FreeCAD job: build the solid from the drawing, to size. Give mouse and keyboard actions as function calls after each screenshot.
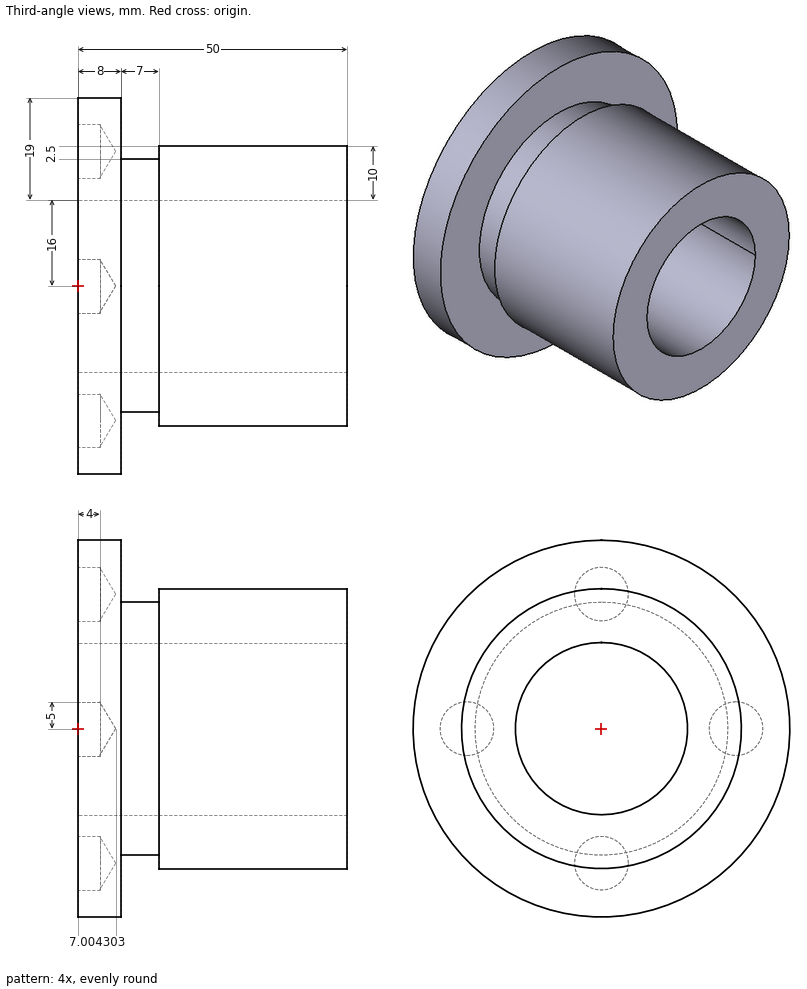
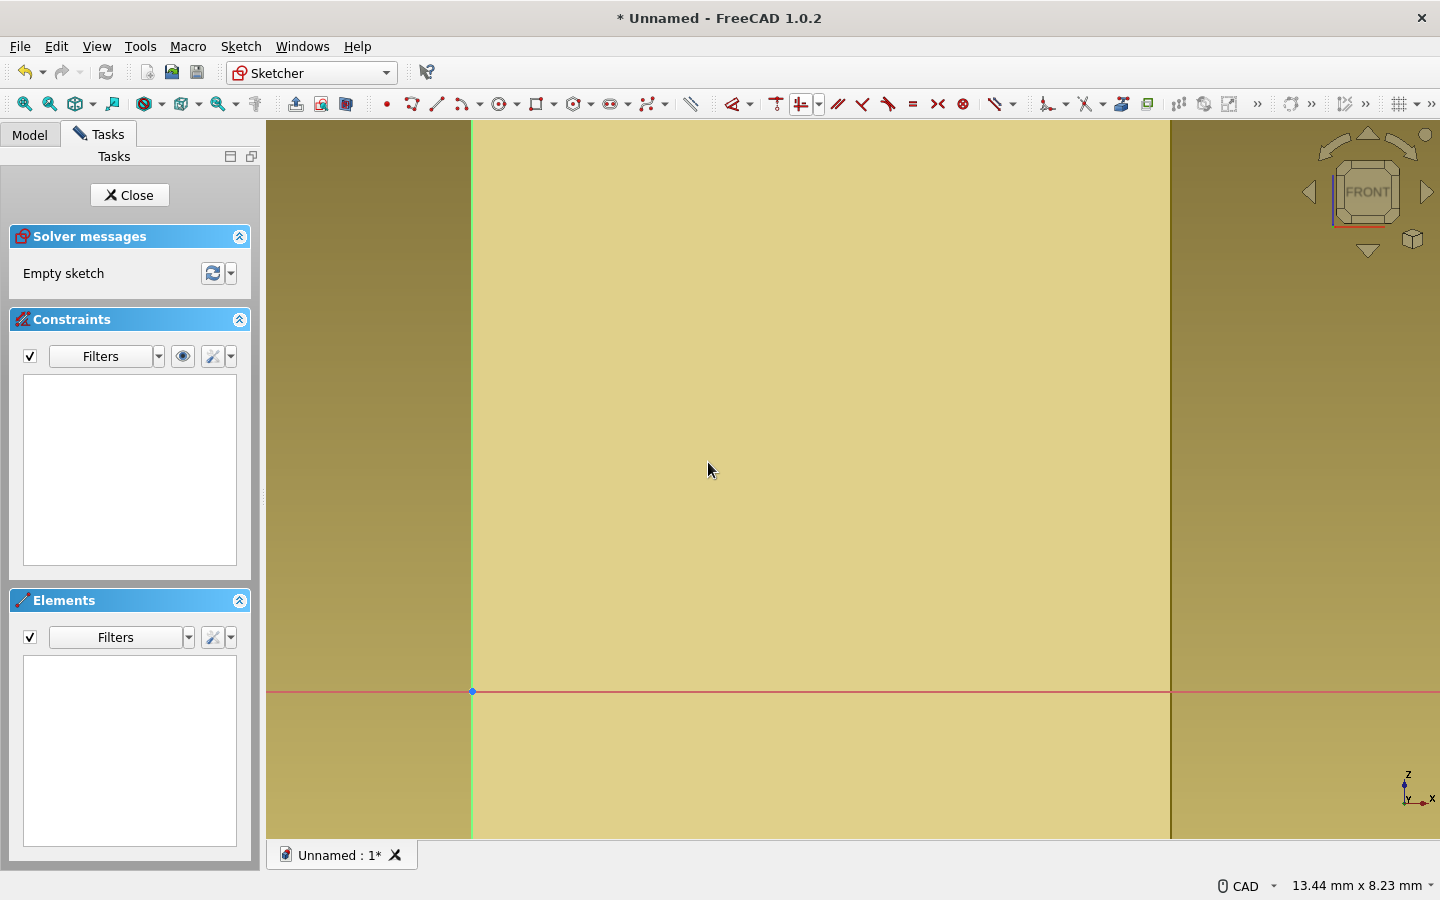
key(g)
key(m)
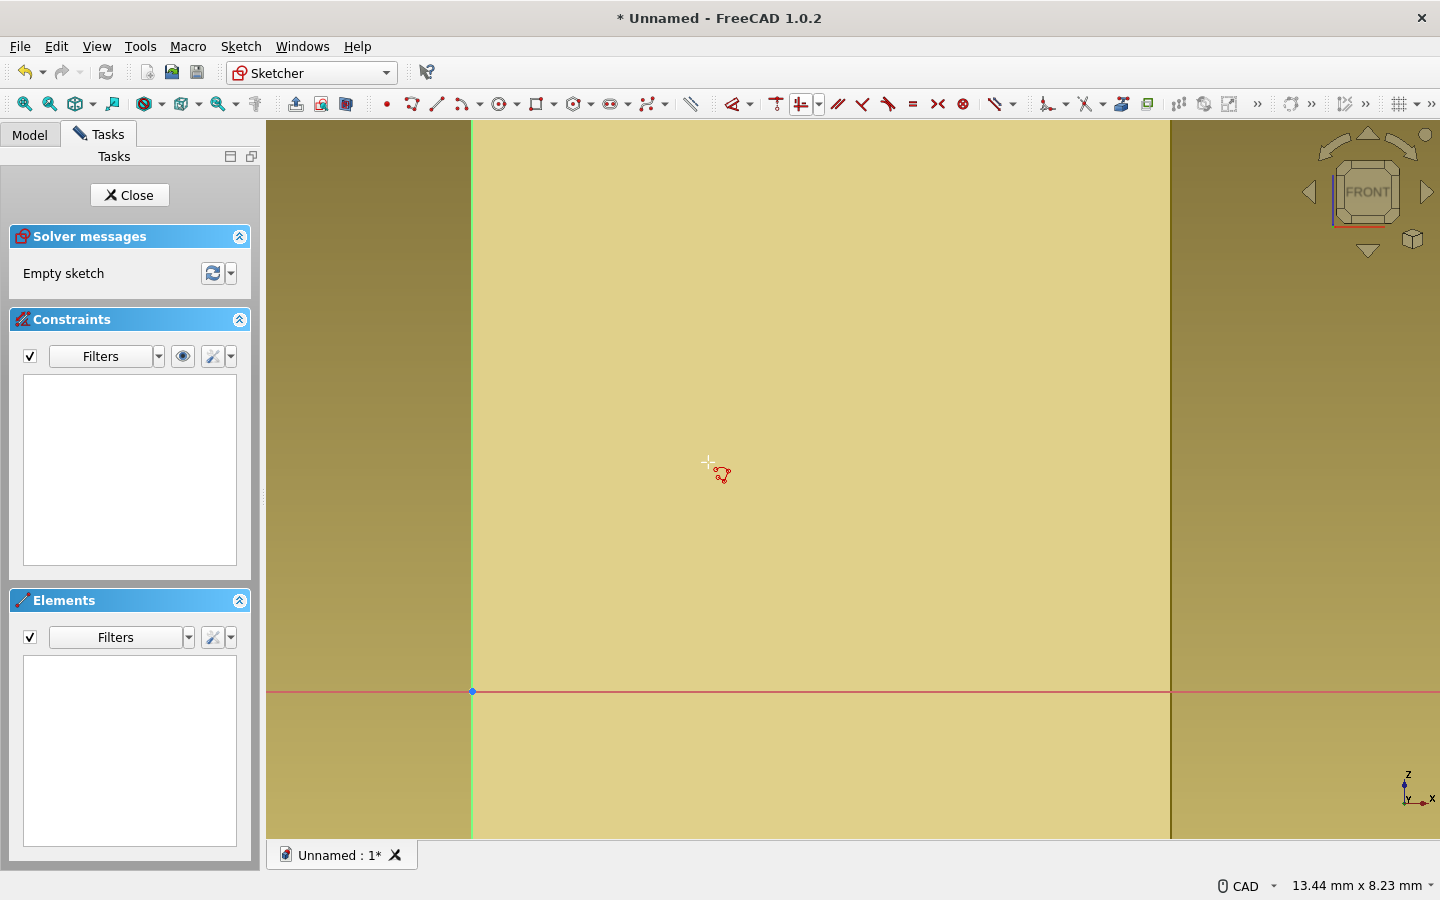
click(472, 692)
click(481, 255)
click(822, 255)
click(1084, 683)
click(472, 692)
key(Escape)
key(Escape)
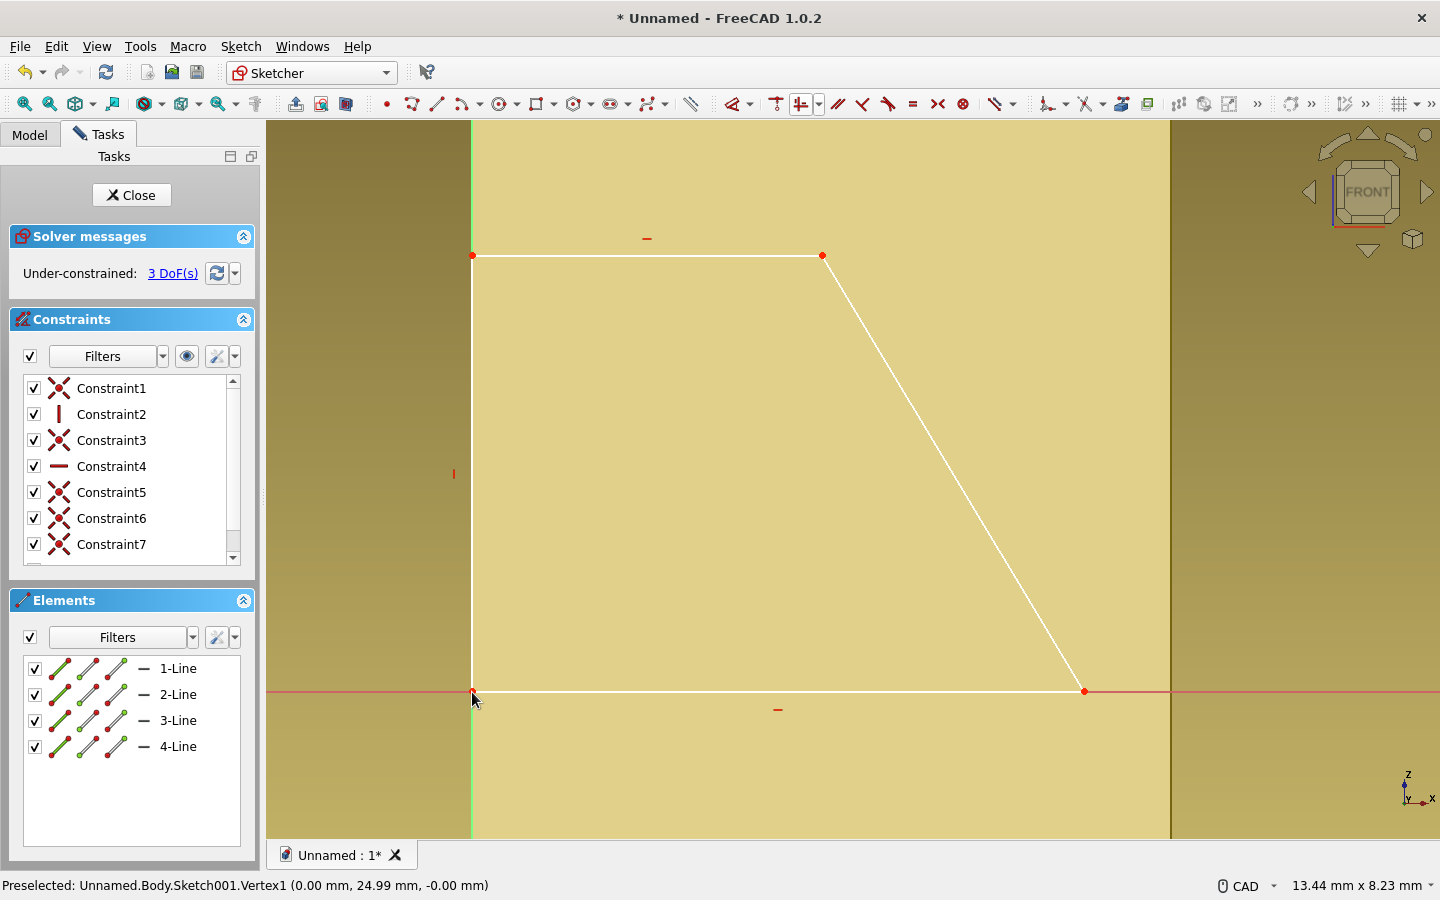
key(d)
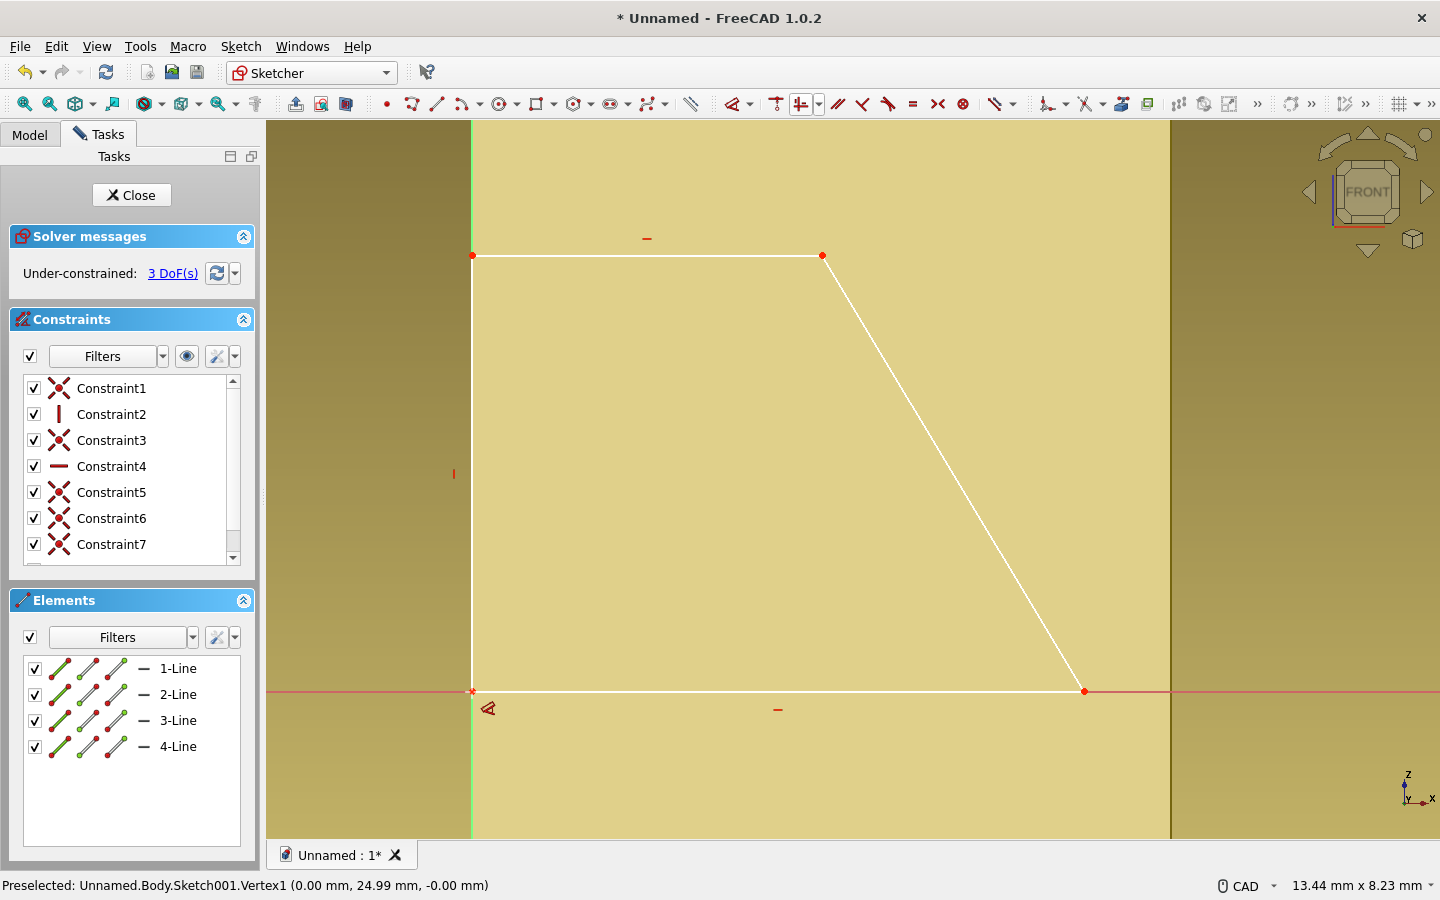
click(472, 561)
click(438, 474)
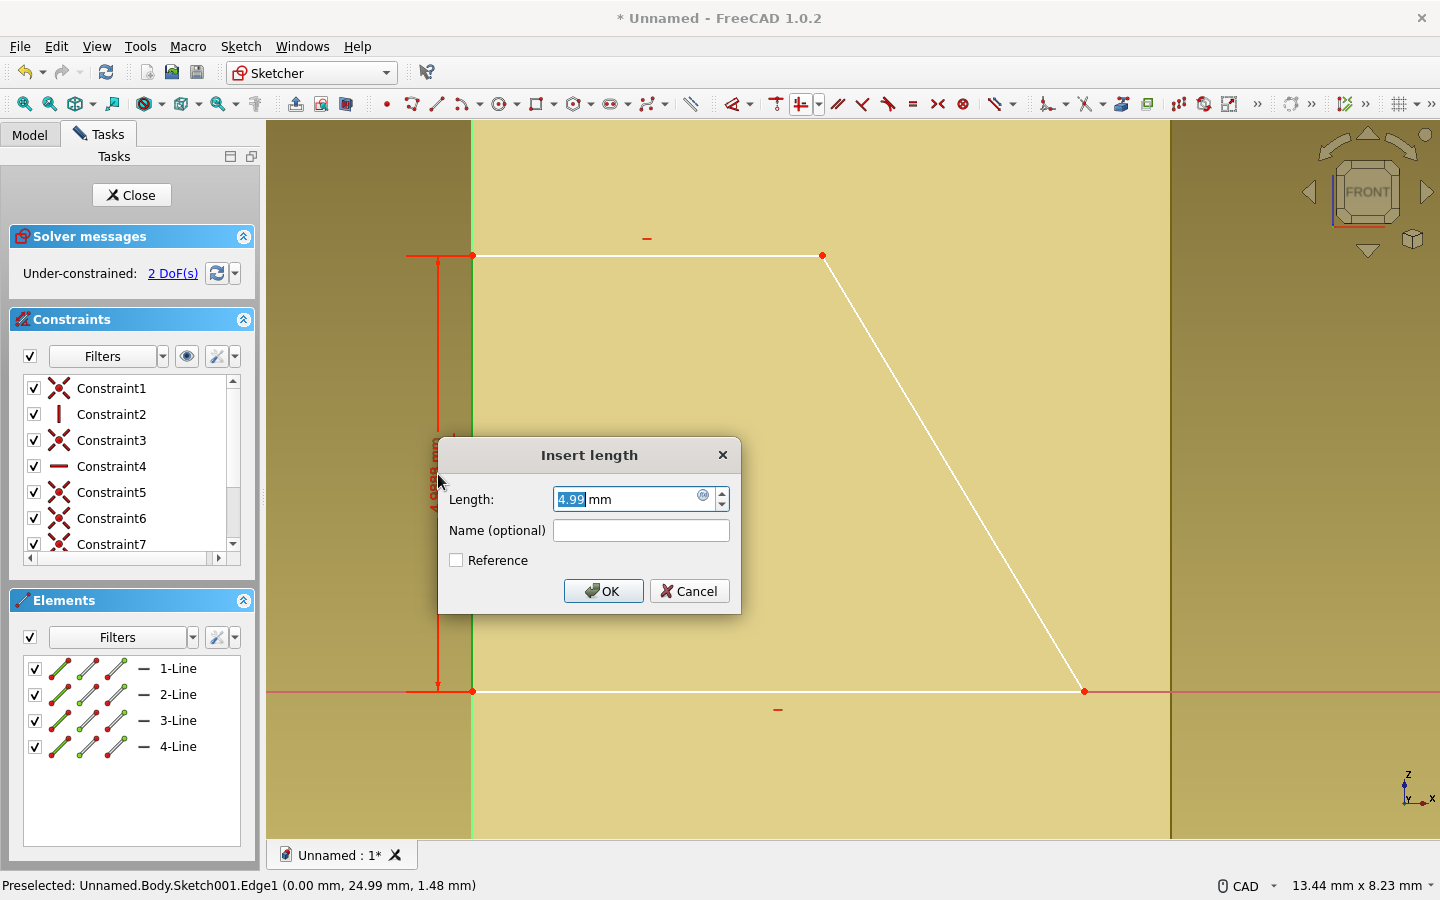
text(5)
key(Return)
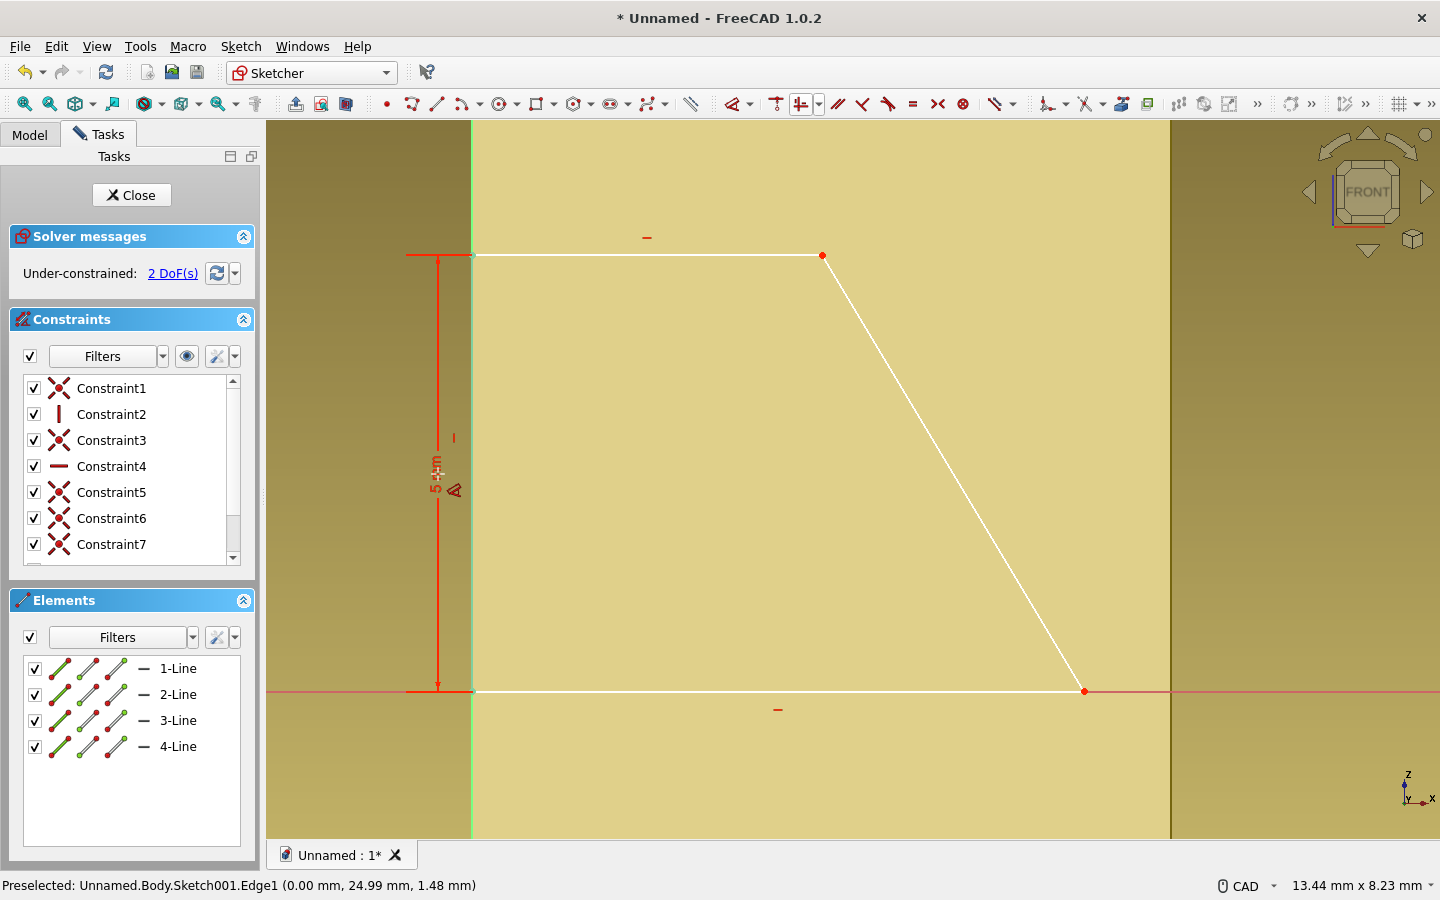
click(577, 255)
click(647, 221)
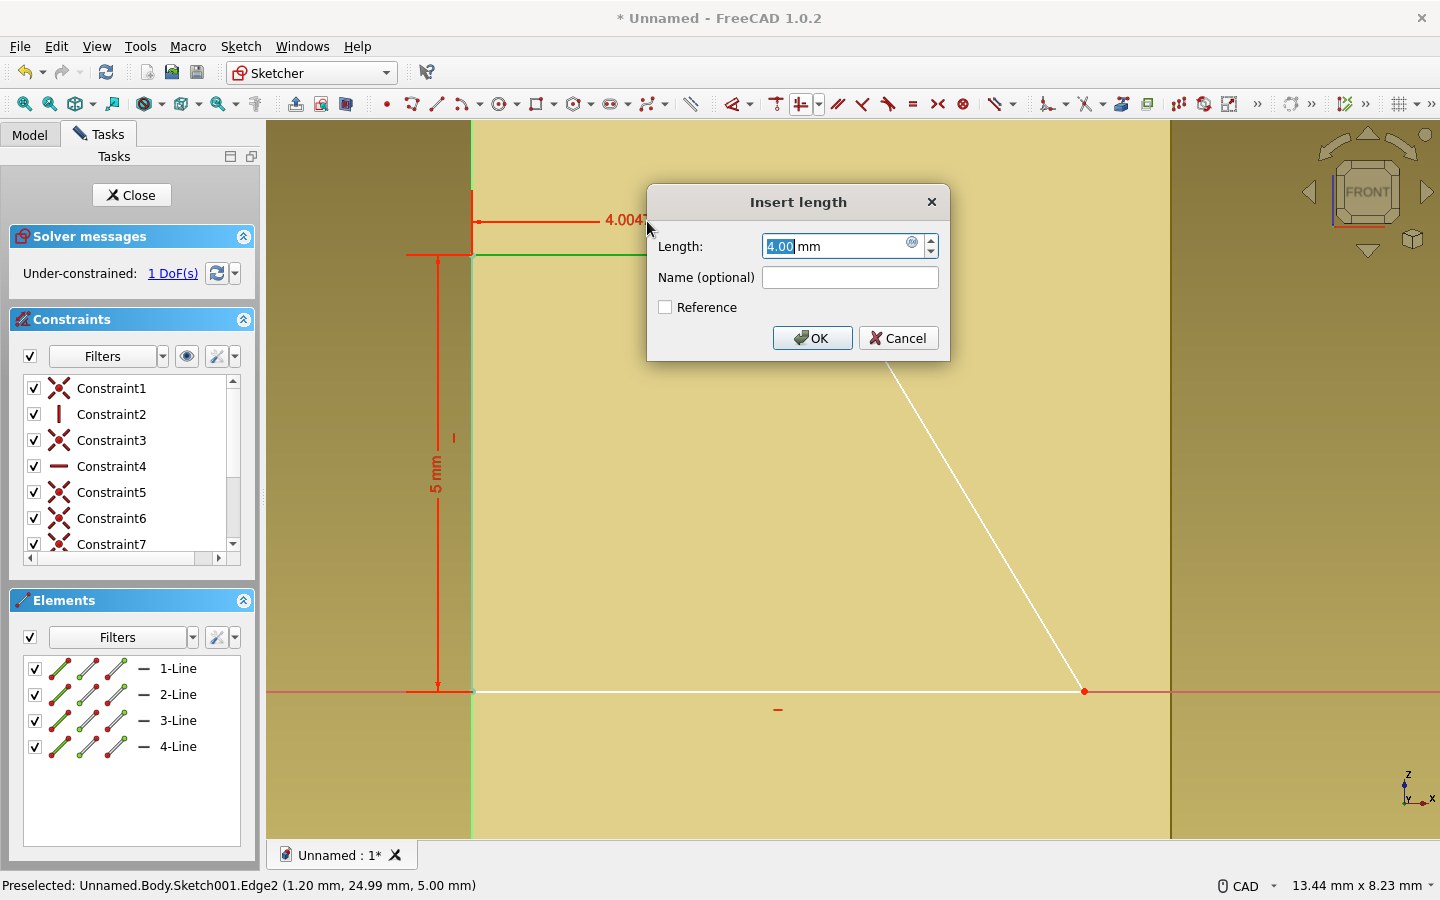
text(4)
key(Return)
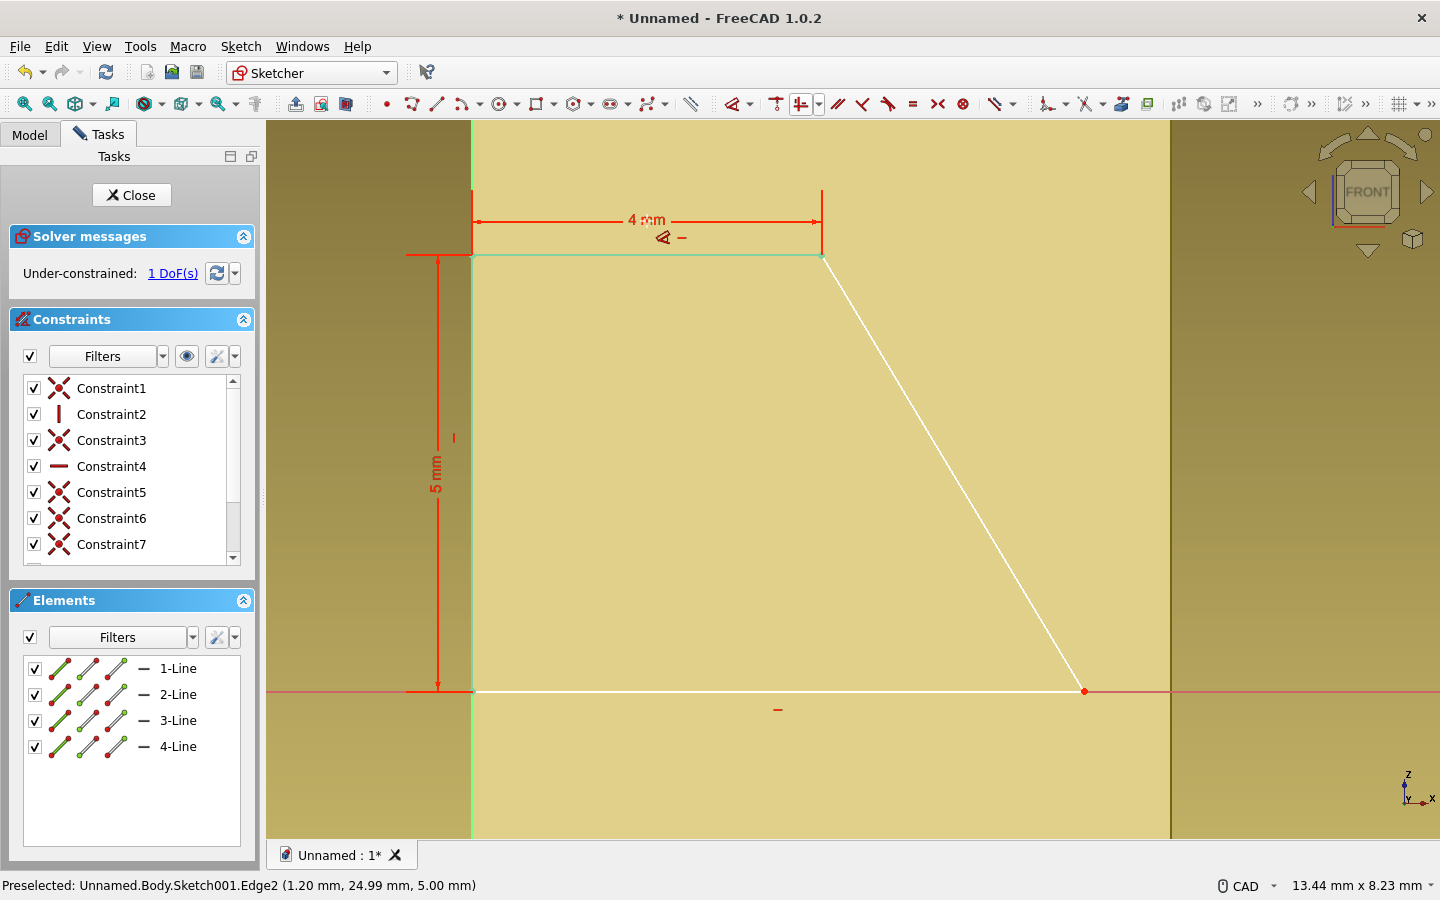
click(900, 692)
click(778, 726)